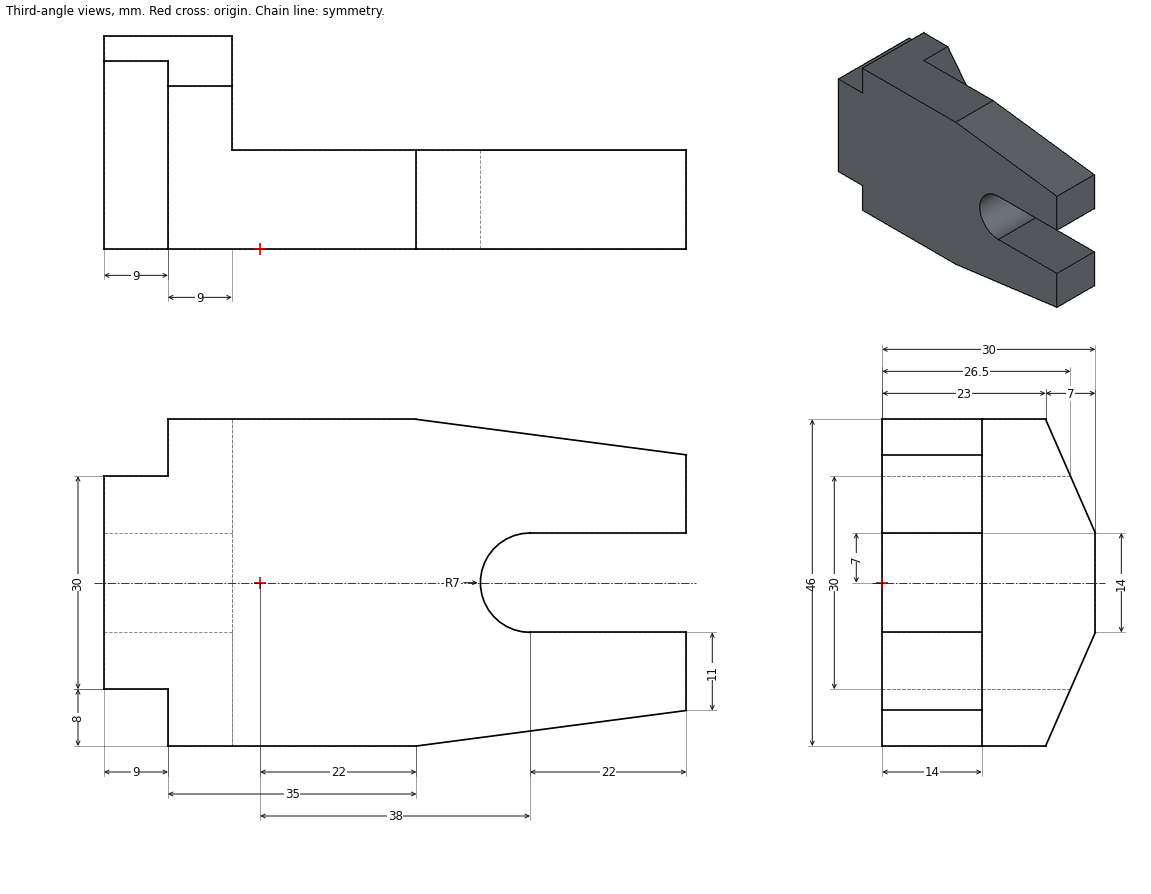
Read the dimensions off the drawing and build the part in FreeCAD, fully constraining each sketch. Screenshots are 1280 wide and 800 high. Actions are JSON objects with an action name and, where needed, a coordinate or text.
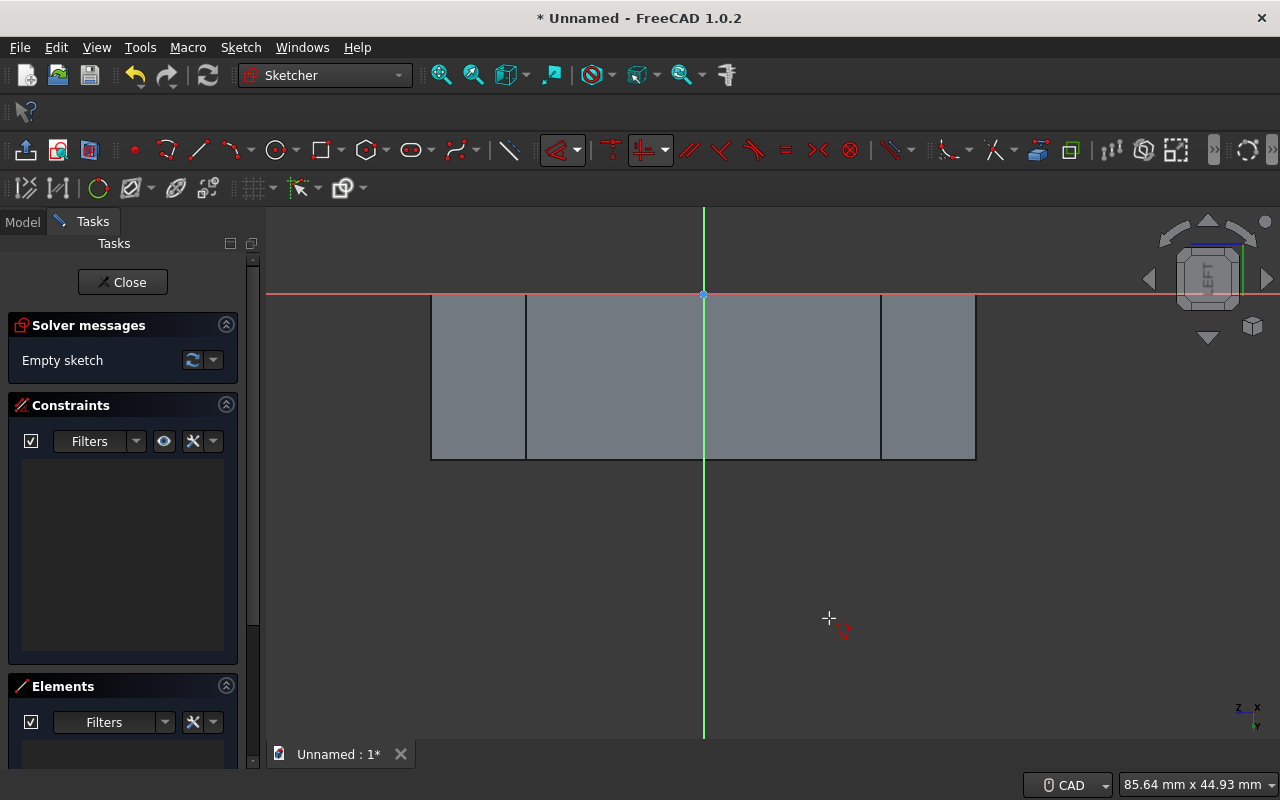
{"action": "left_click", "coordinate": [881, 294]}
{"action": "left_click", "coordinate": [526, 303]}
{"action": "left_click", "coordinate": [526, 608]}
{"action": "left_click", "coordinate": [621, 650]}
{"action": "left_click", "coordinate": [787, 650]}
{"action": "left_click", "coordinate": [881, 608]}
{"action": "left_click", "coordinate": [881, 294]}
{"action": "key", "text": "Escape"}
{"action": "key", "text": "Escape"}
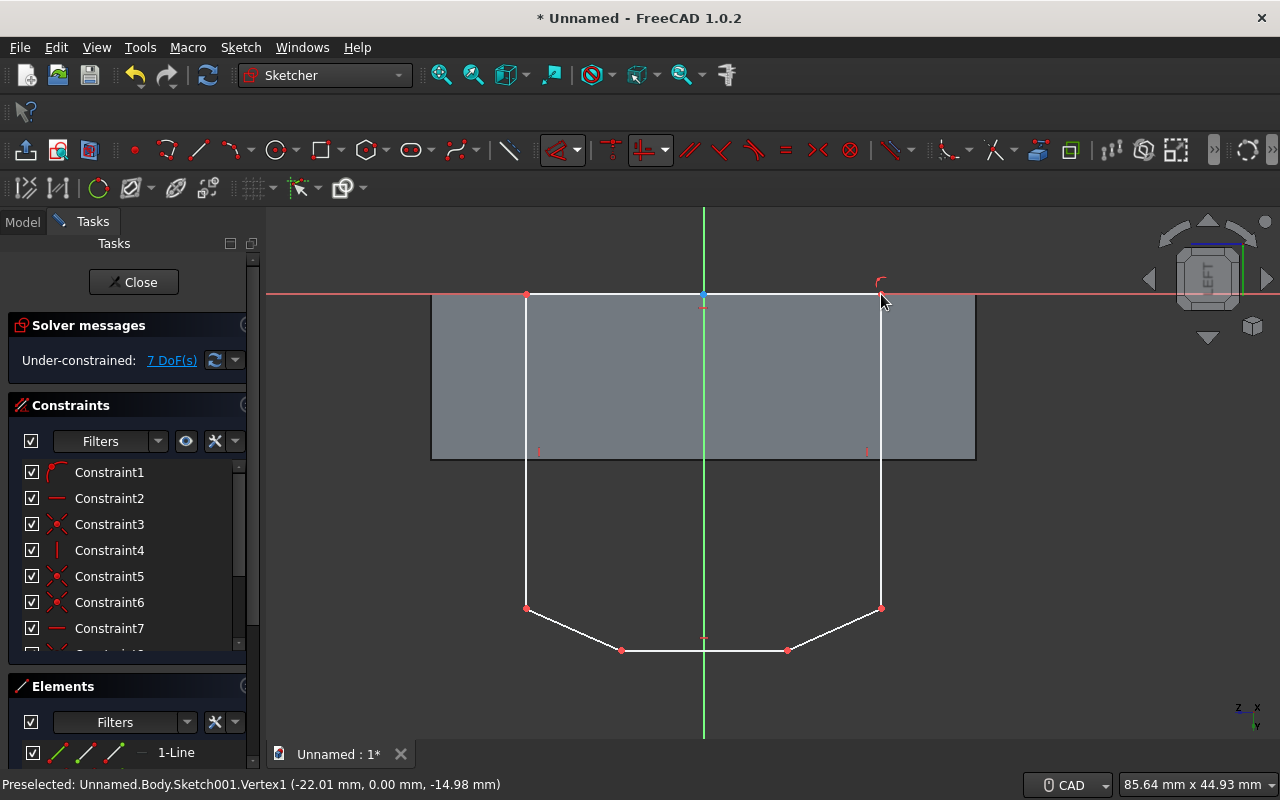
{"action": "left_click", "coordinate": [526, 609]}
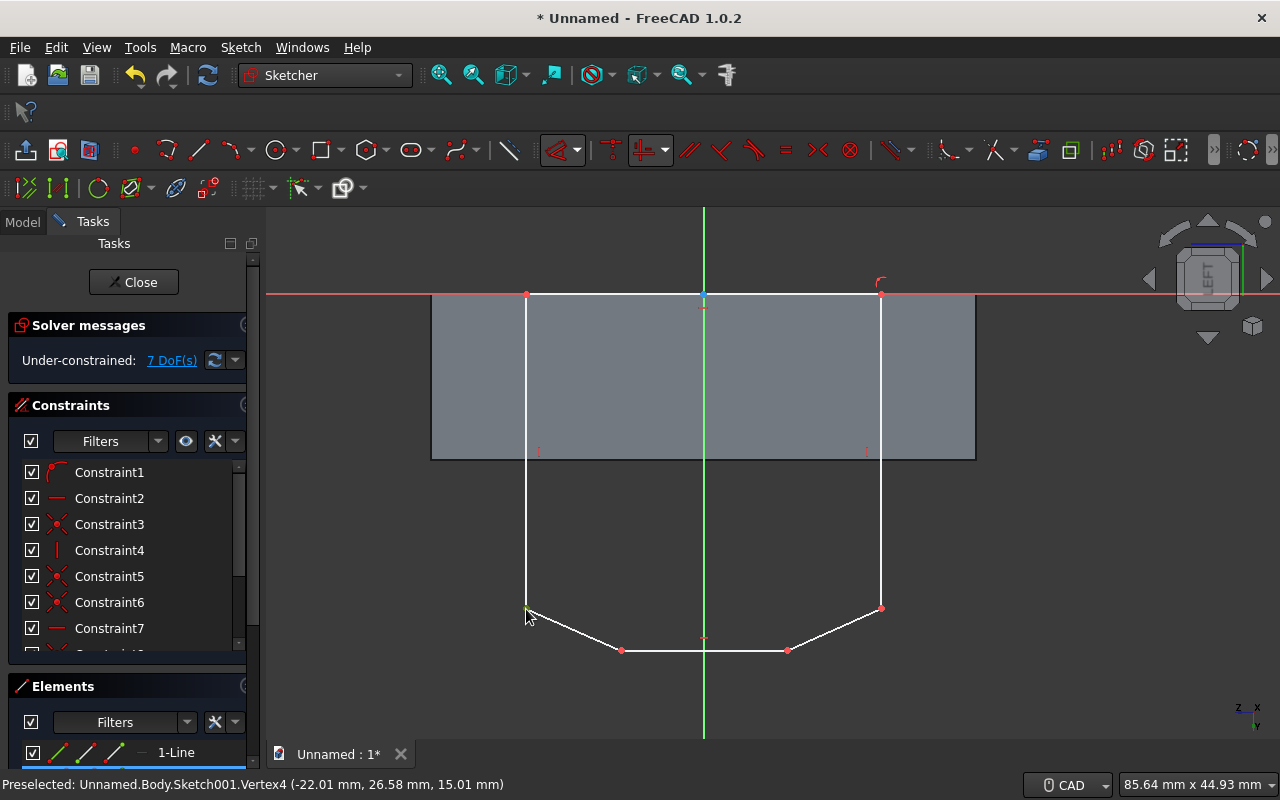
{"action": "left_click", "coordinate": [881, 609]}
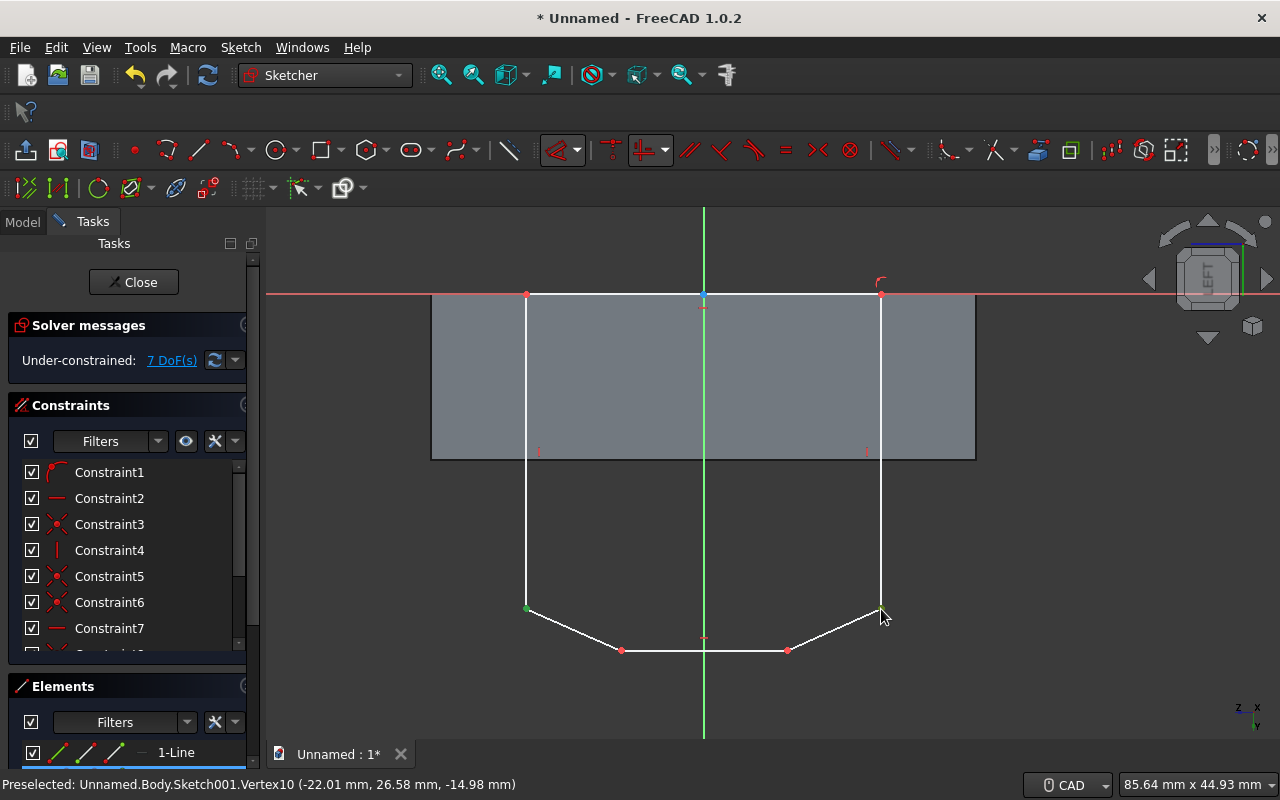
{"action": "left_click", "coordinate": [704, 609]}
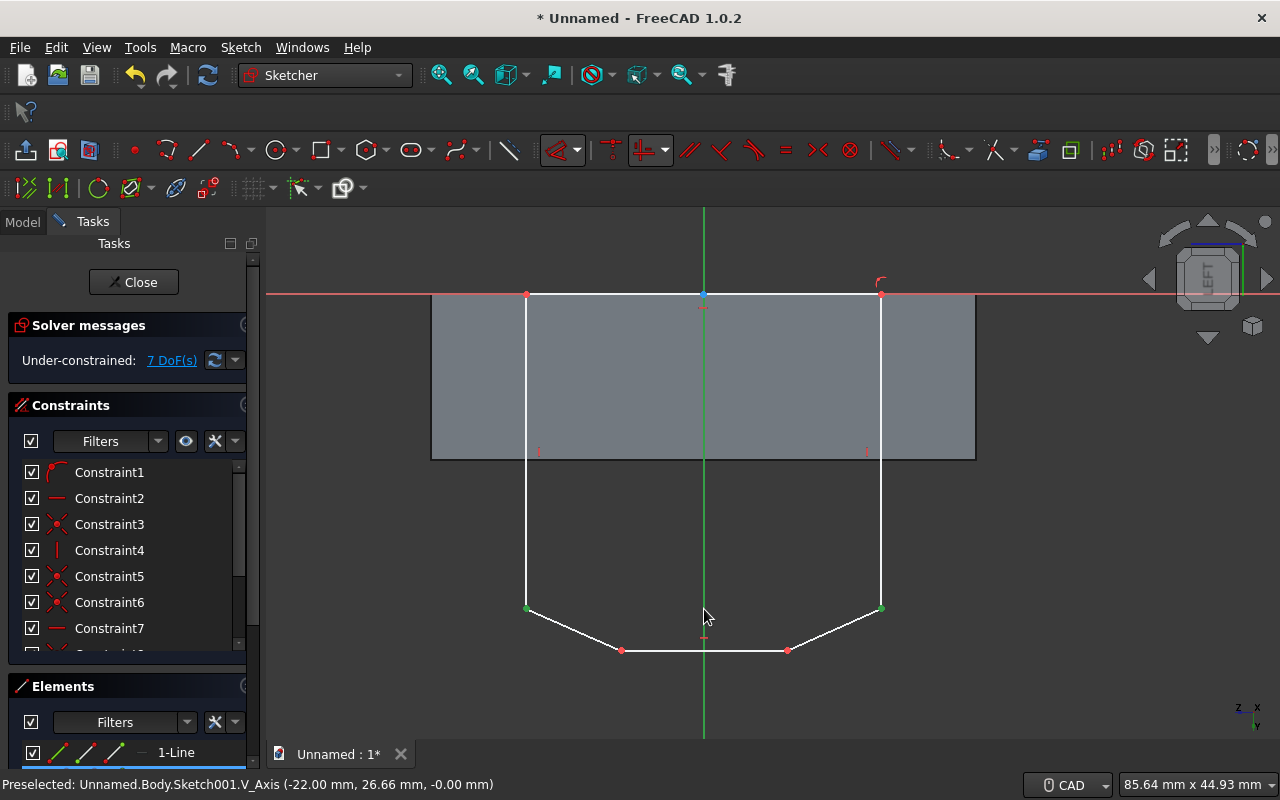
{"action": "left_click", "coordinate": [818, 150]}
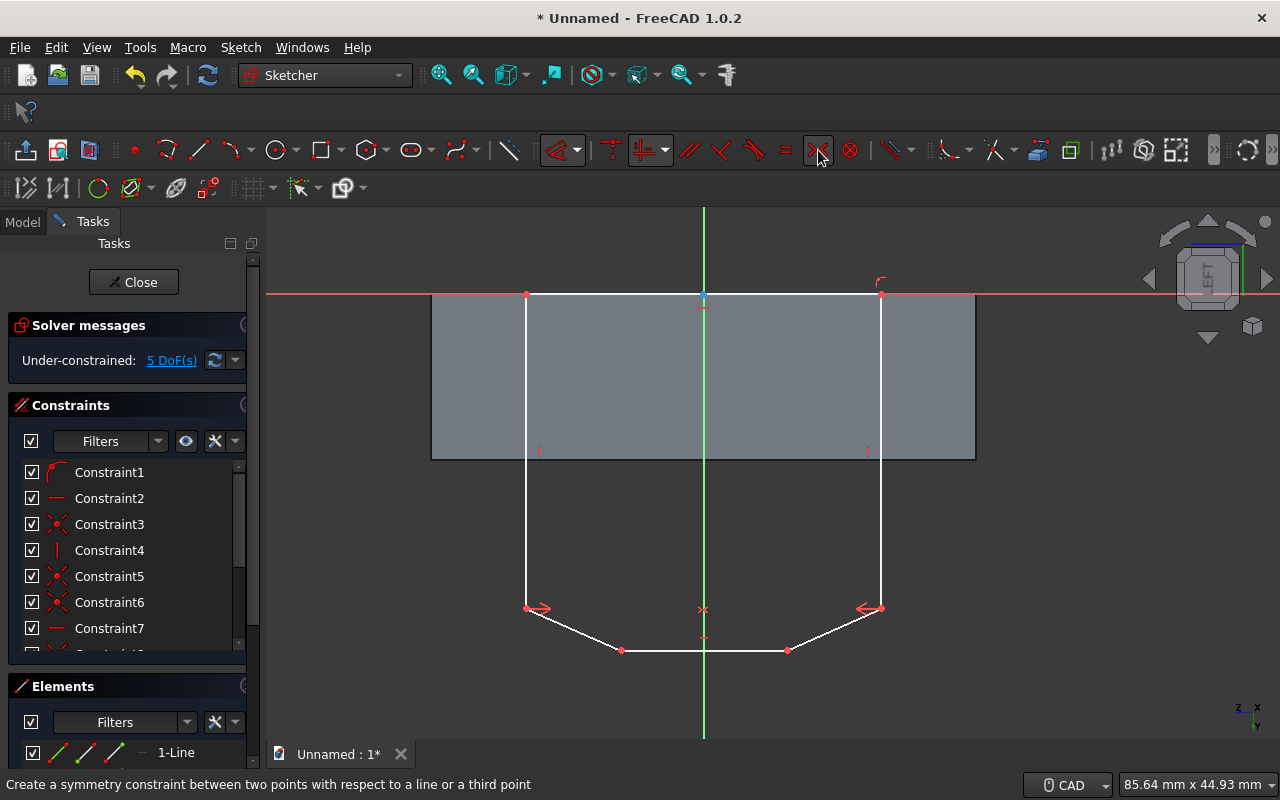
{"action": "key", "text": "d"}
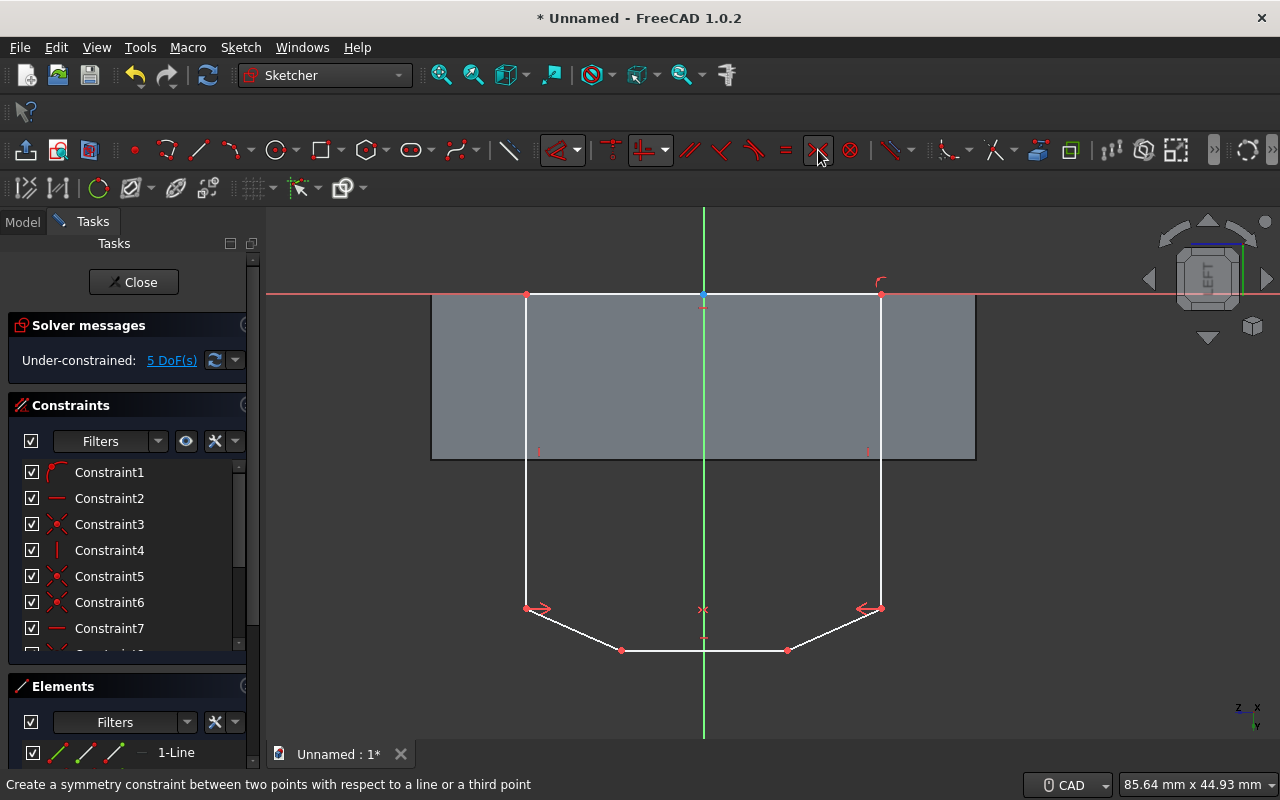
{"action": "left_click", "coordinate": [775, 294]}
{"action": "left_click", "coordinate": [622, 260]}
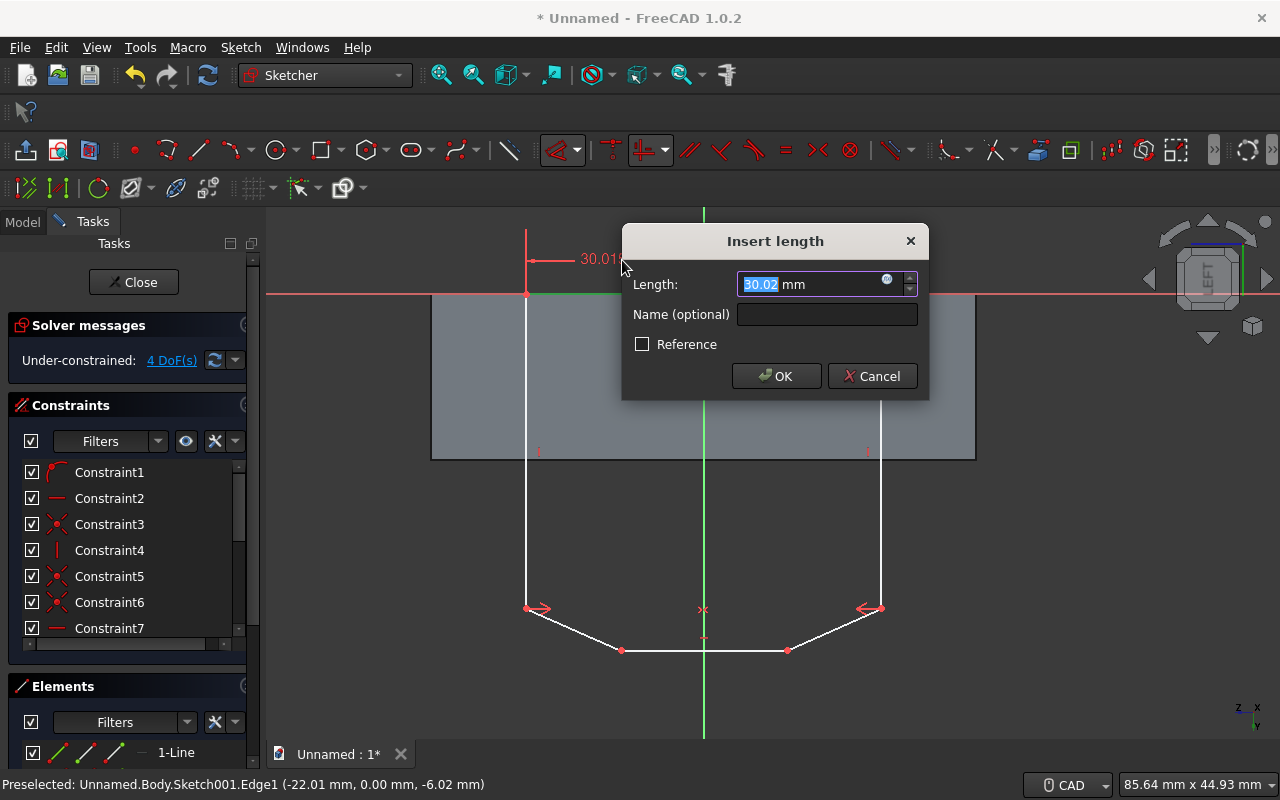
{"action": "type", "text": "30"}
{"action": "key", "text": "Return"}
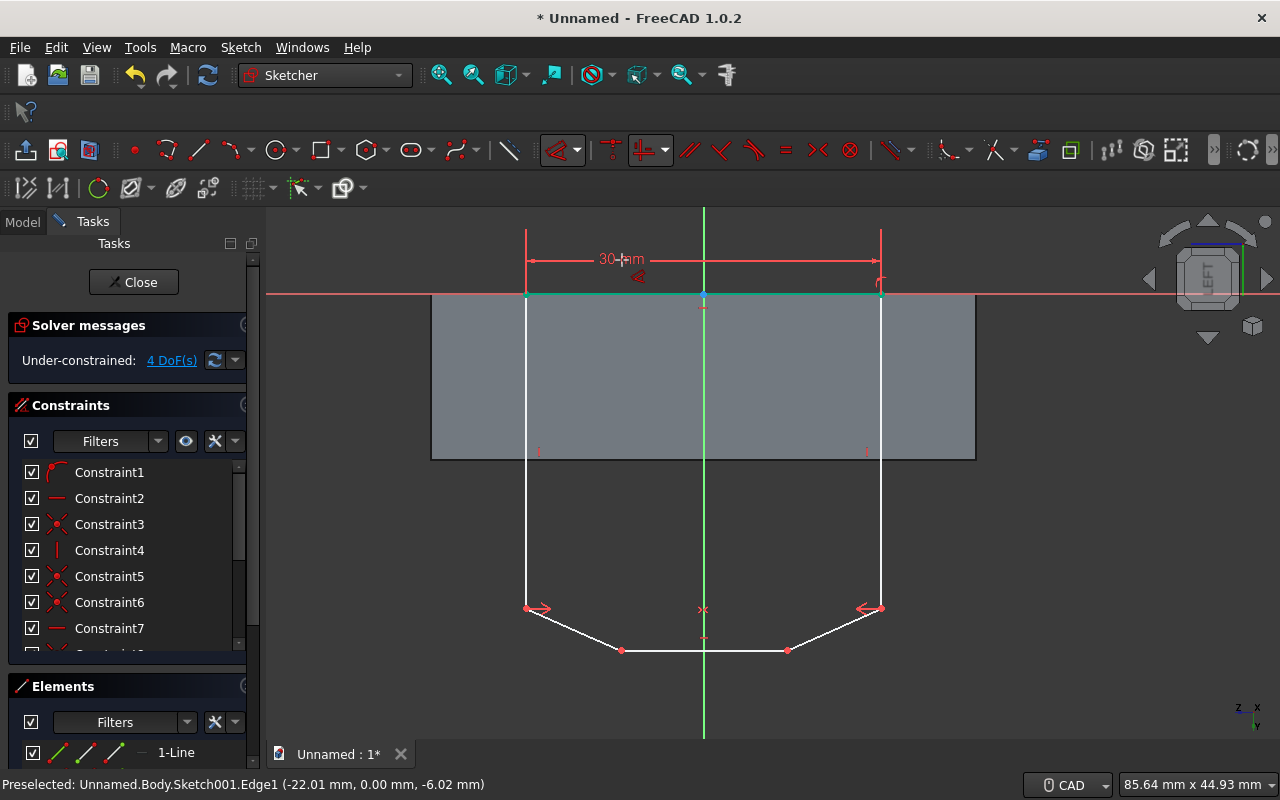
{"action": "left_click", "coordinate": [671, 651]}
{"action": "left_click", "coordinate": [666, 685]}